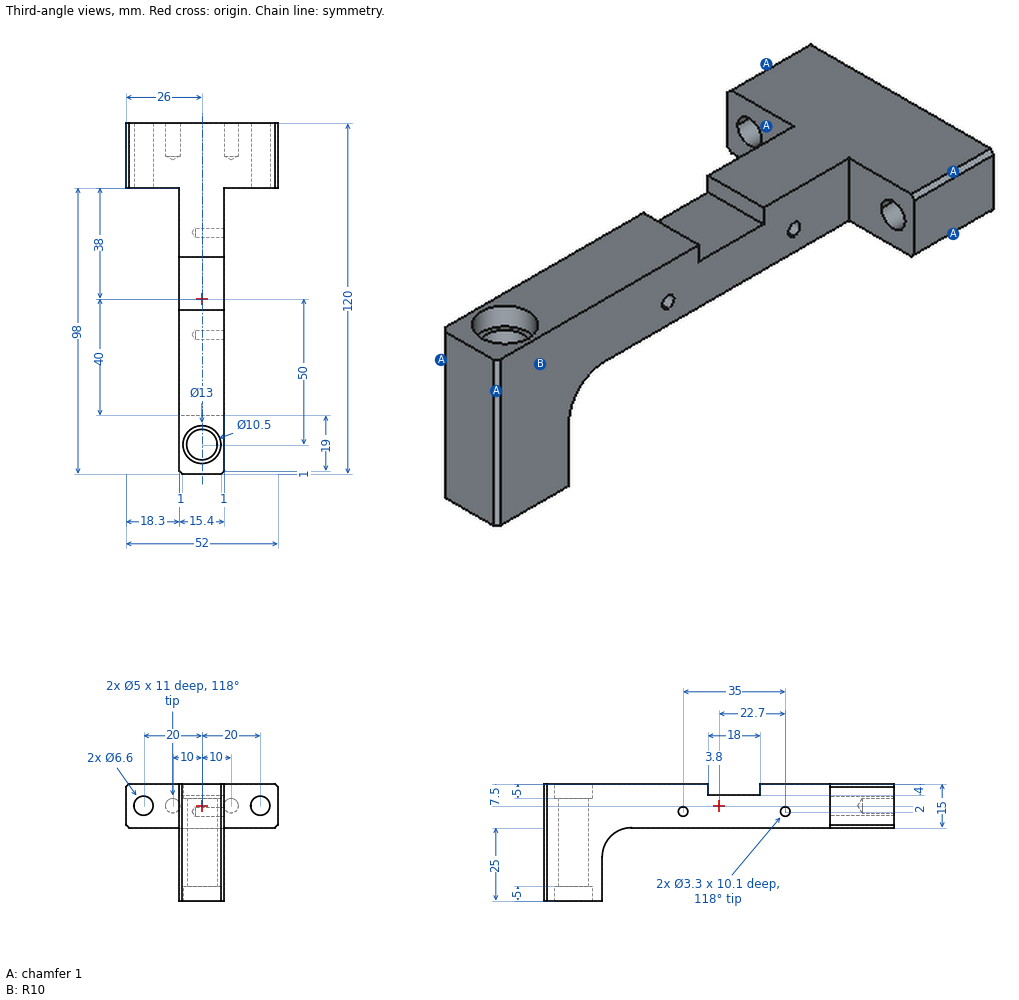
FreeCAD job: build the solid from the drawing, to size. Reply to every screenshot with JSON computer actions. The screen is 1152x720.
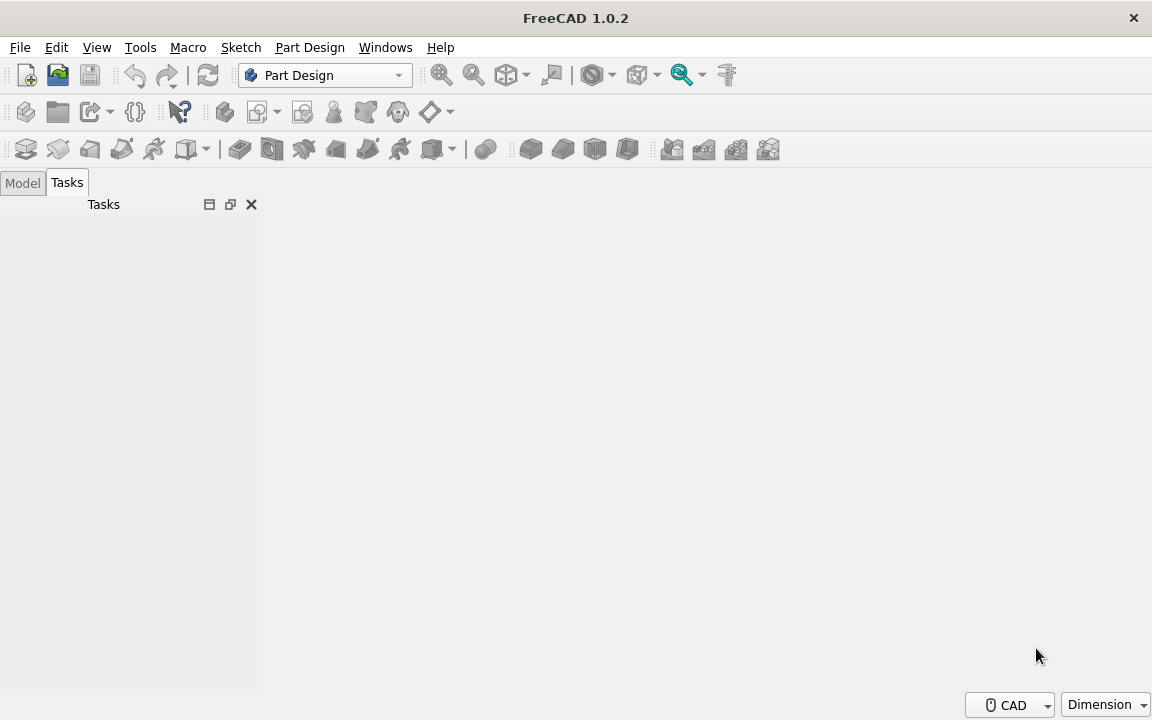
{"action": "left_click", "coordinate": [26, 76]}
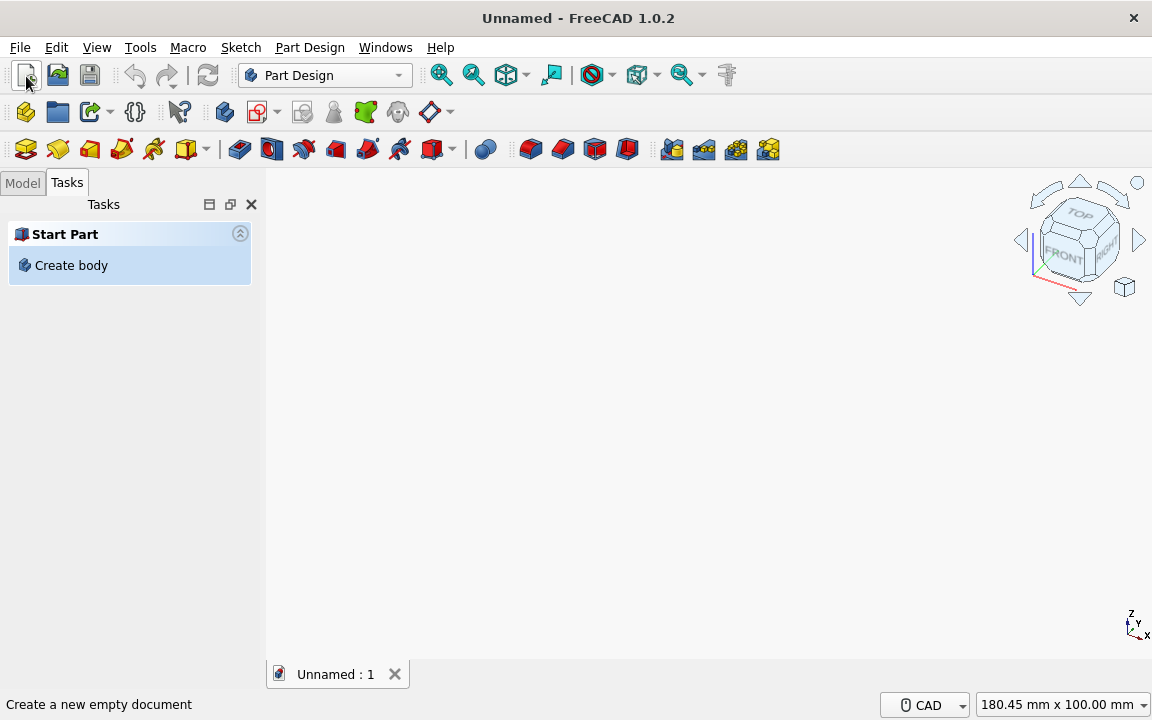
{"action": "left_click", "coordinate": [258, 112]}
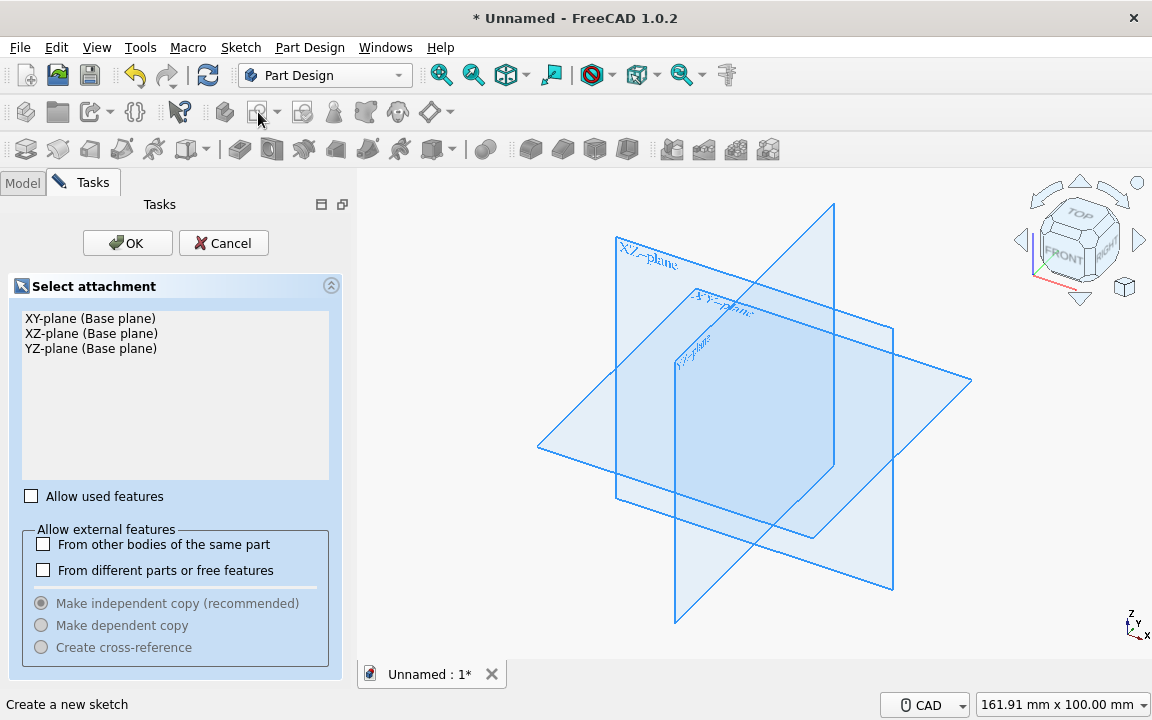
{"action": "left_click", "coordinate": [82, 318]}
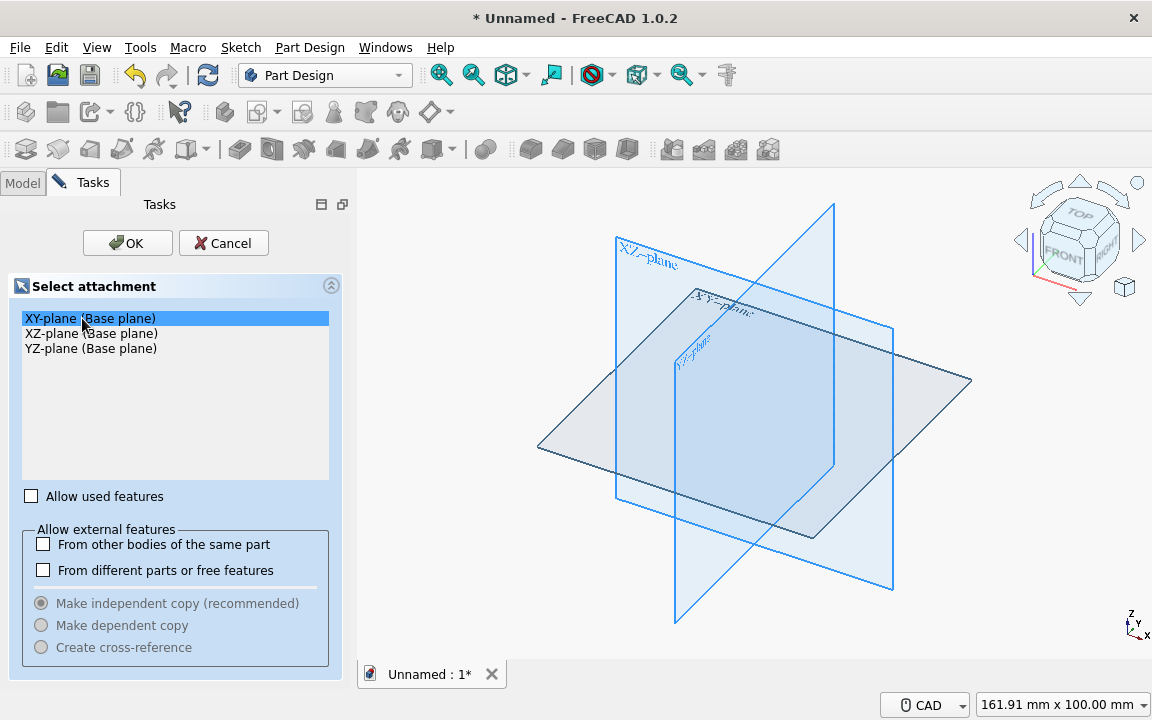
{"action": "left_click", "coordinate": [128, 243]}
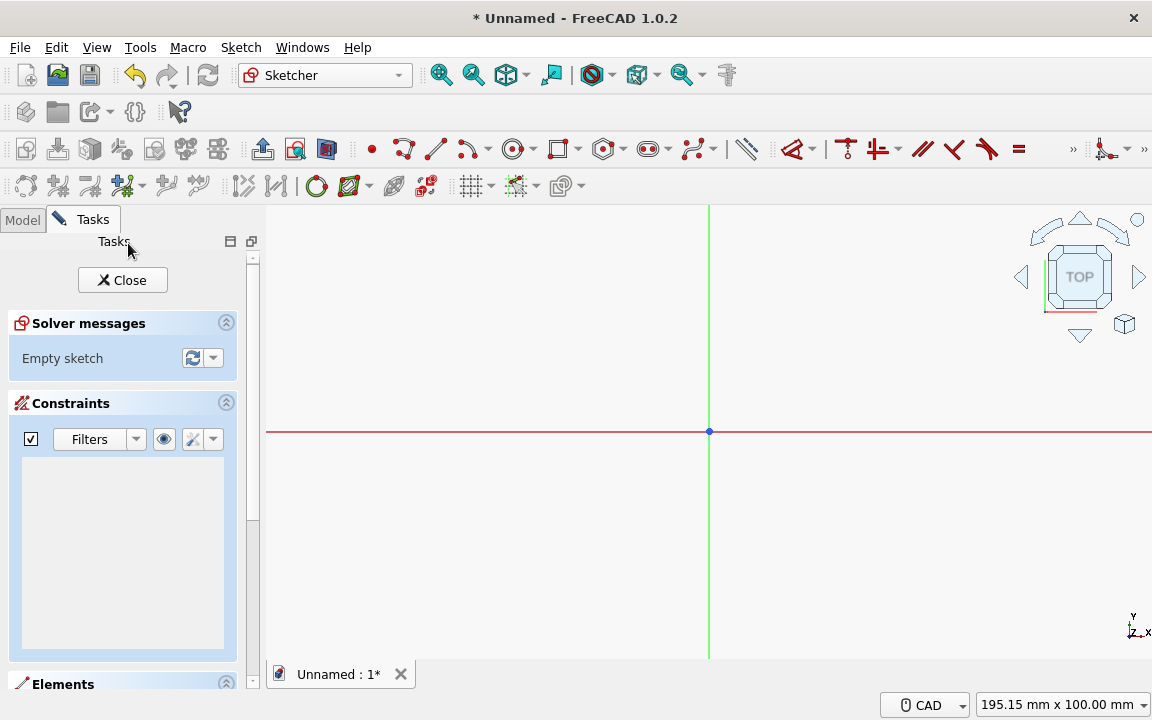
{"action": "scroll", "coordinate": [557, 432], "scroll_direction": "down", "scroll_amount": 3}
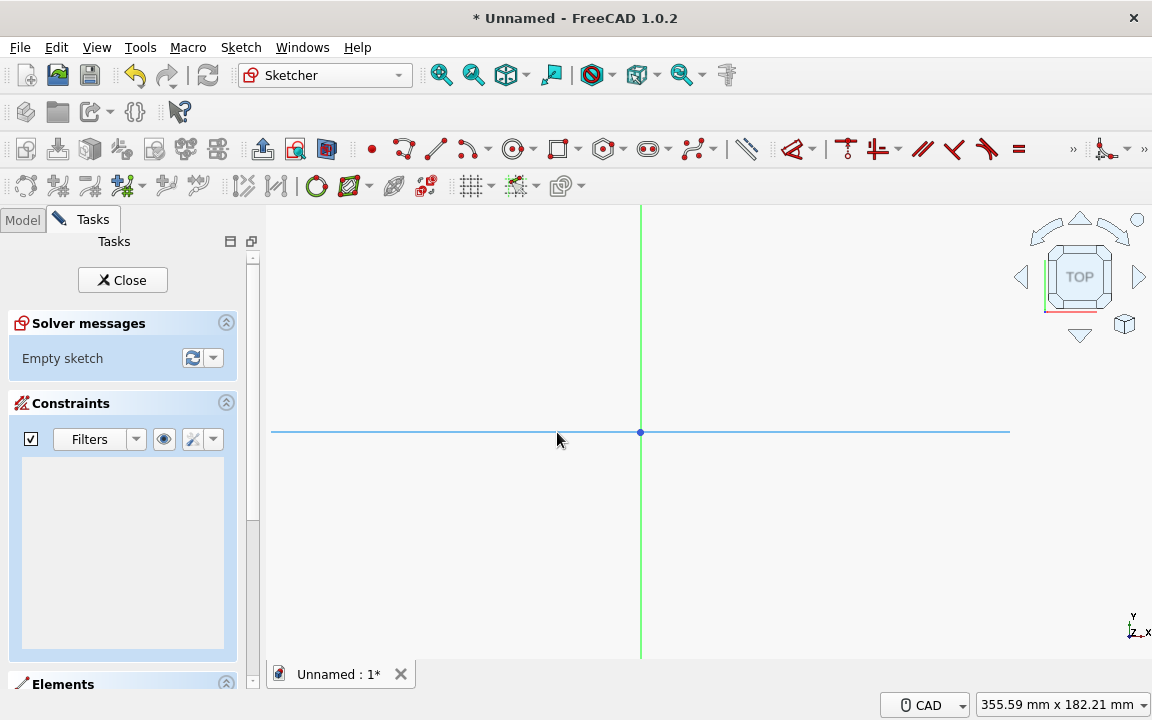
{"action": "key", "text": "g v"}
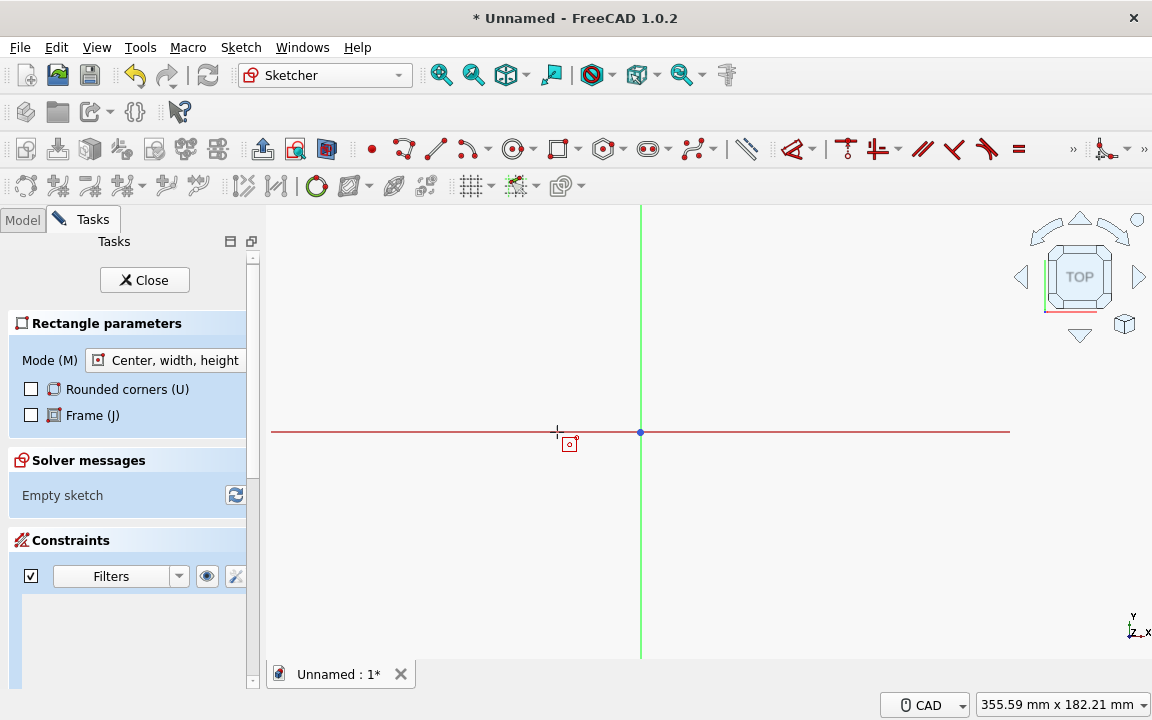
{"action": "left_click", "coordinate": [641, 432]}
{"action": "mouse_move", "coordinate": [705, 283]}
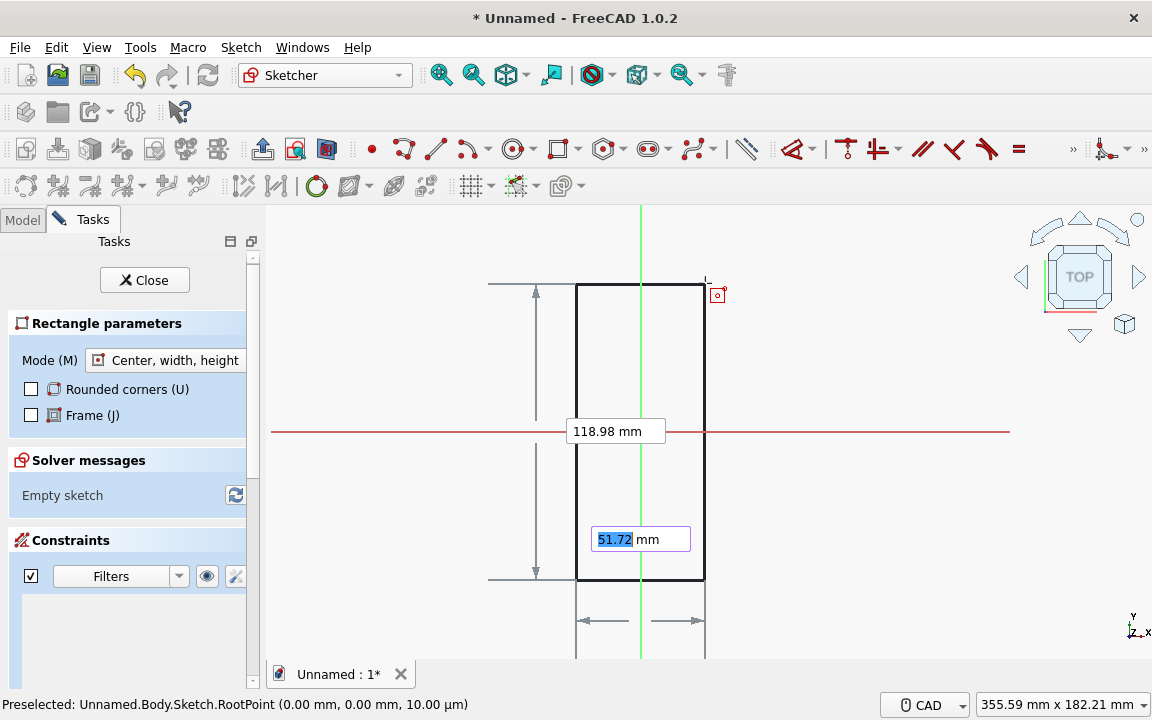
{"action": "type", "text": "52"}
{"action": "key", "text": "Tab"}
{"action": "type", "text": "120"}
{"action": "key", "text": "Return"}
{"action": "key", "text": "Escape"}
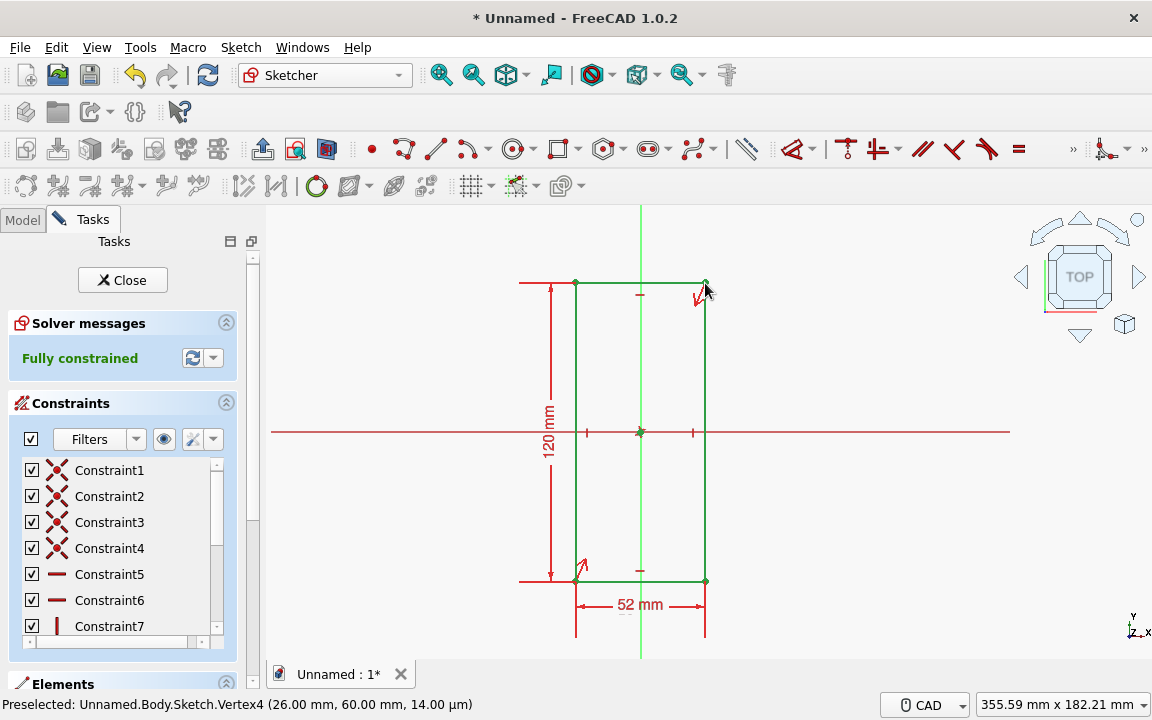
{"action": "left_click", "coordinate": [123, 280]}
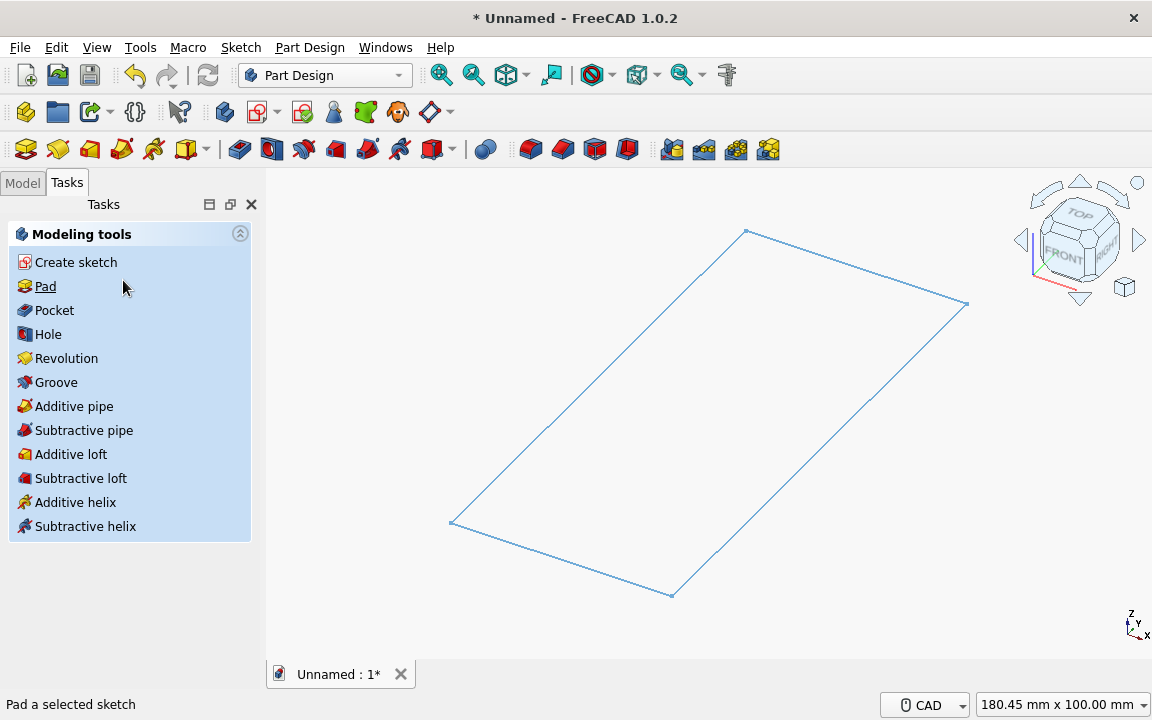
{"action": "left_click", "coordinate": [26, 150]}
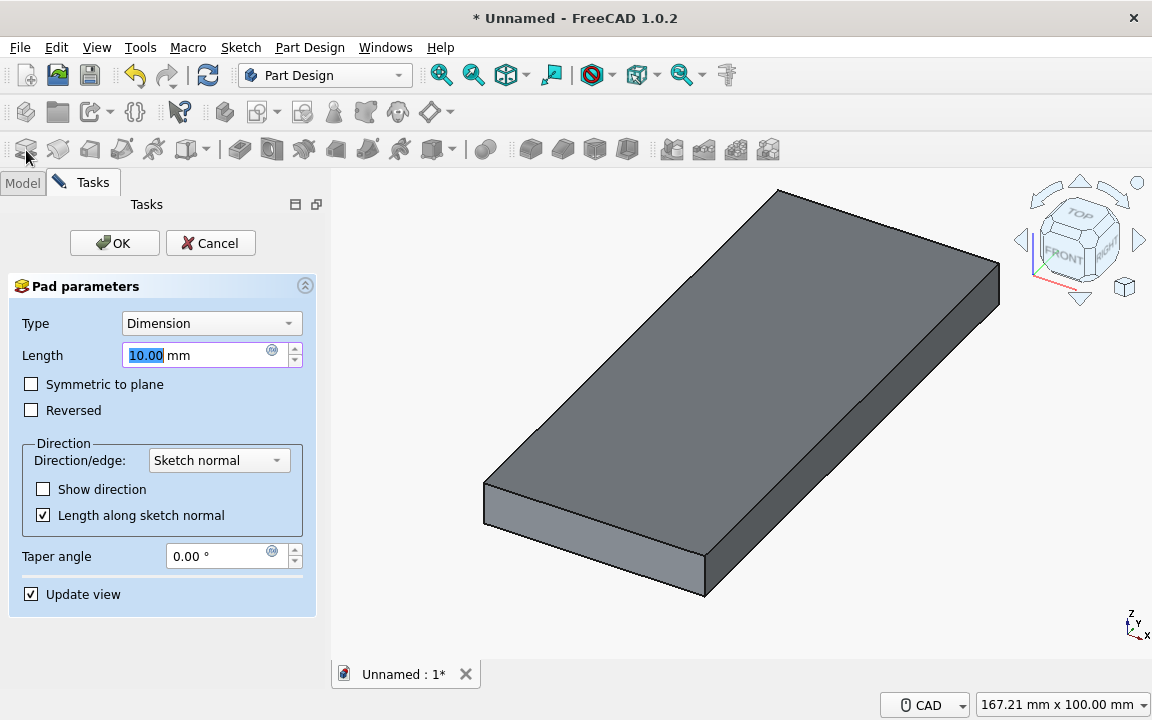
{"action": "type", "text": "15"}
{"action": "key", "text": "Tab"}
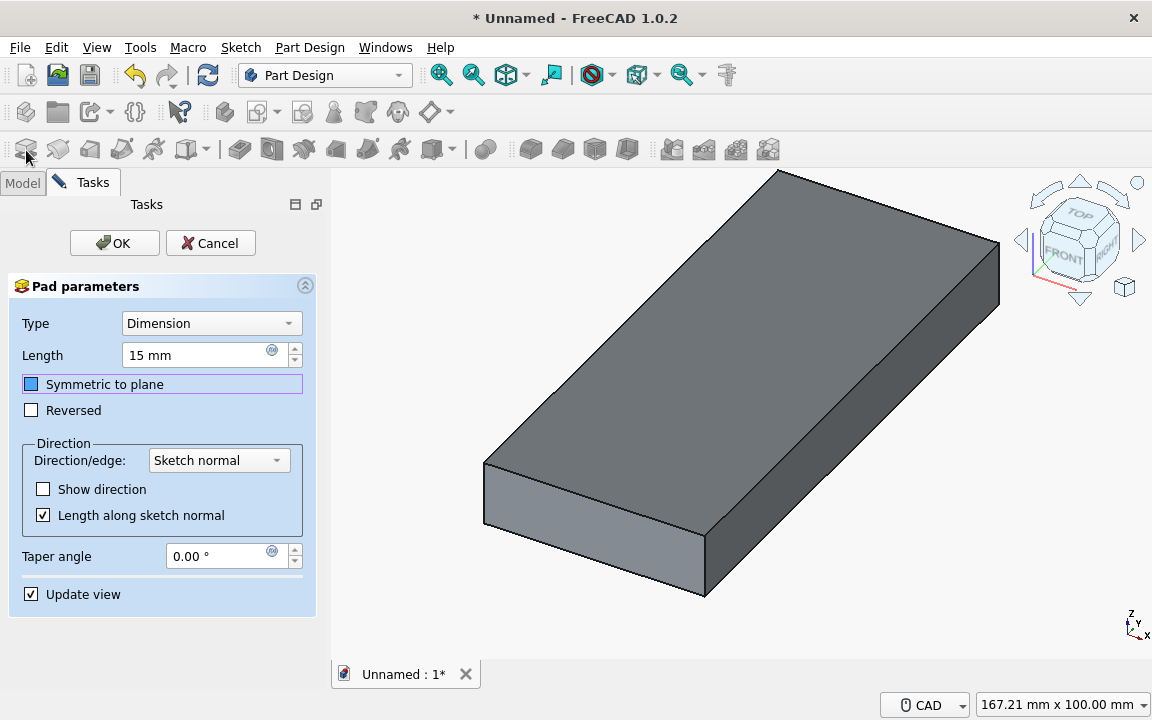
{"action": "left_click", "coordinate": [30, 384]}